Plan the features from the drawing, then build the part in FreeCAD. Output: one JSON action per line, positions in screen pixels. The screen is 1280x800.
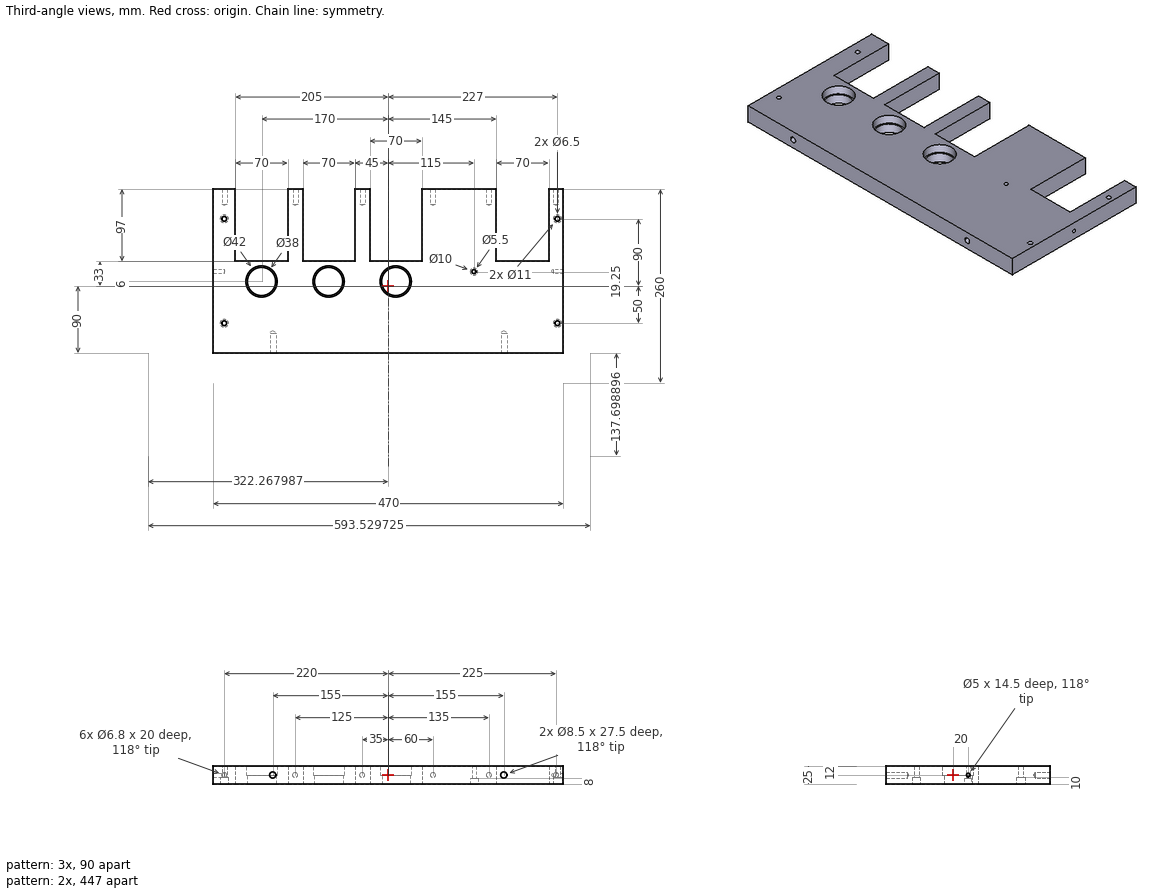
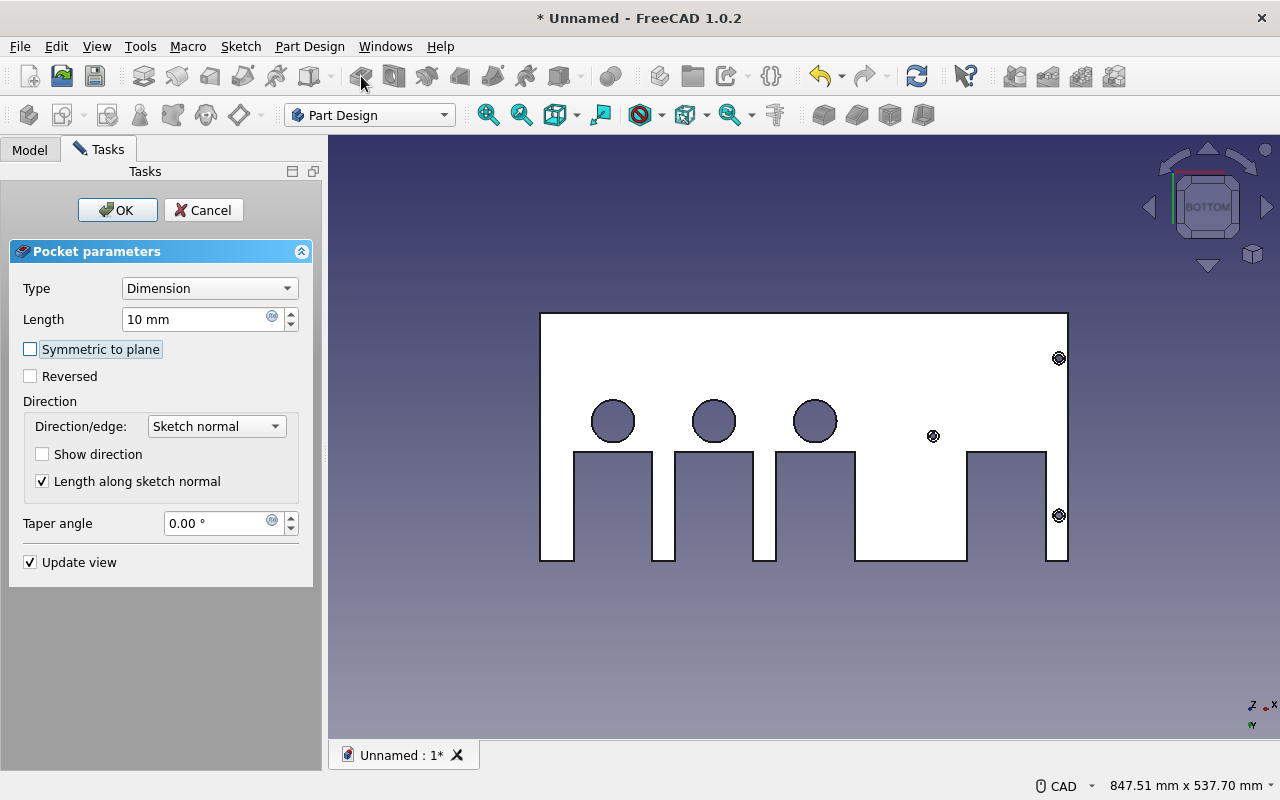
{"action": "left_click", "coordinate": [118, 210]}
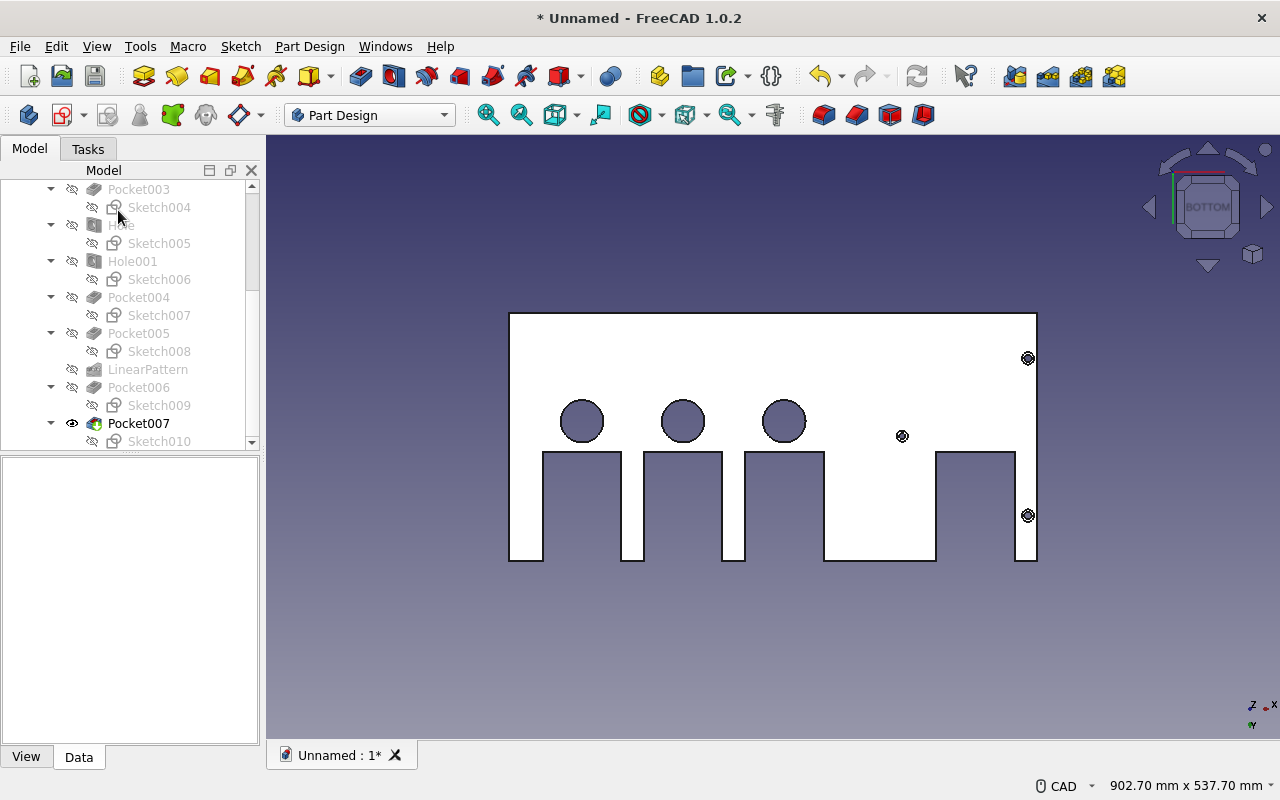
{"action": "left_click", "coordinate": [117, 387]}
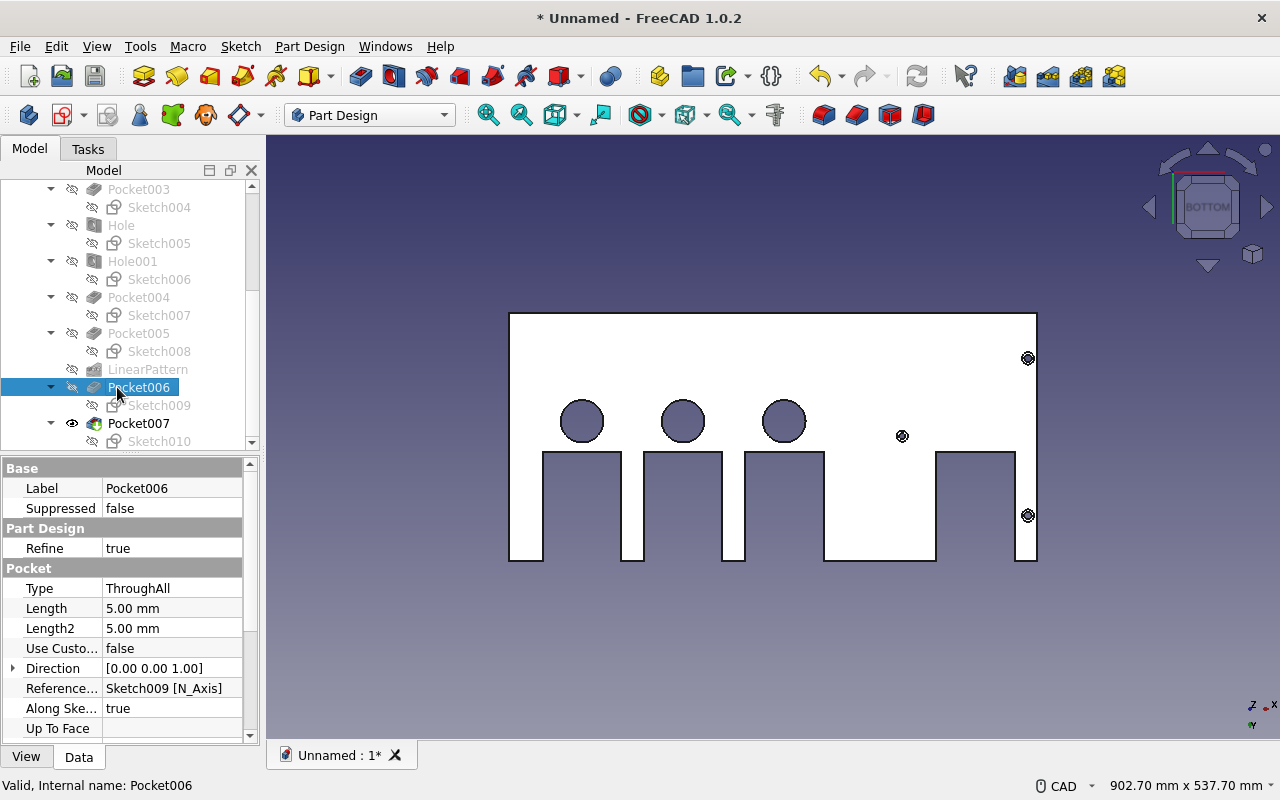
{"action": "left_click", "coordinate": [117, 423], "text": "ctrl"}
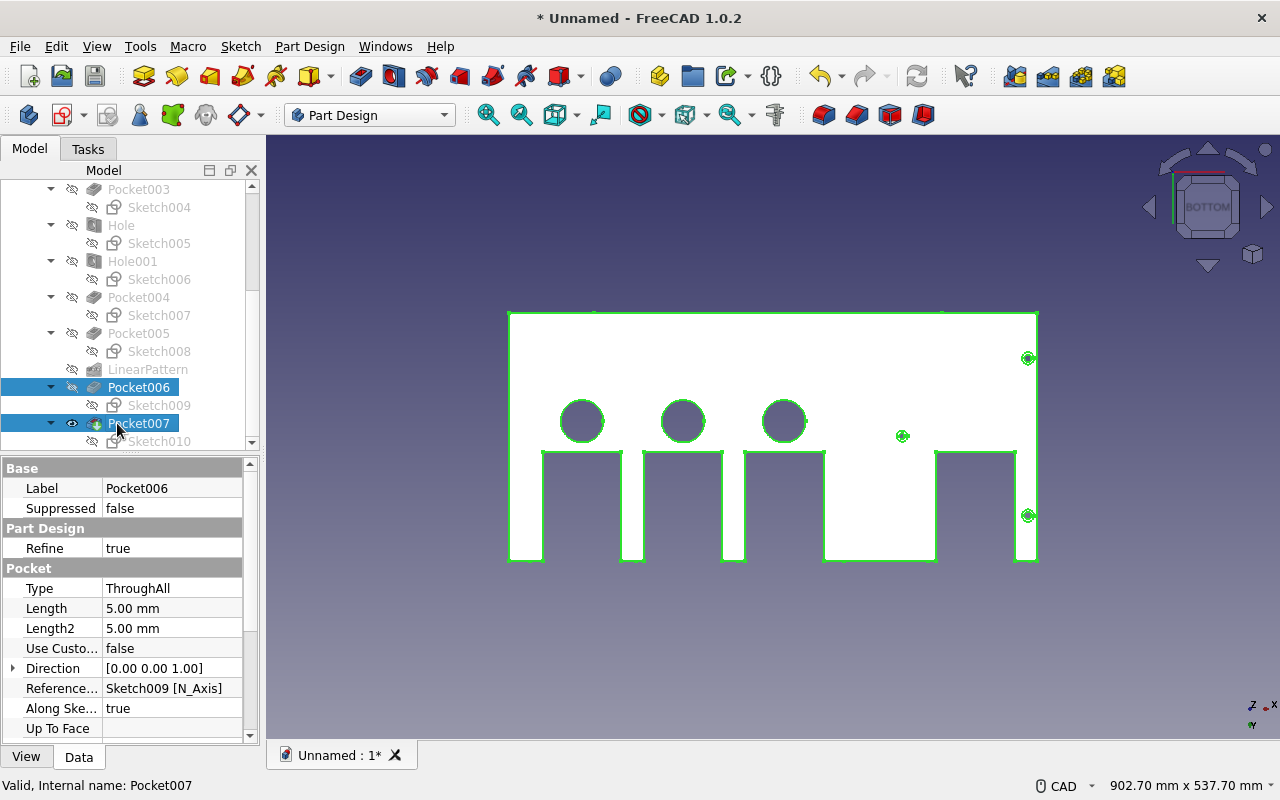
{"action": "left_click", "coordinate": [1048, 76]}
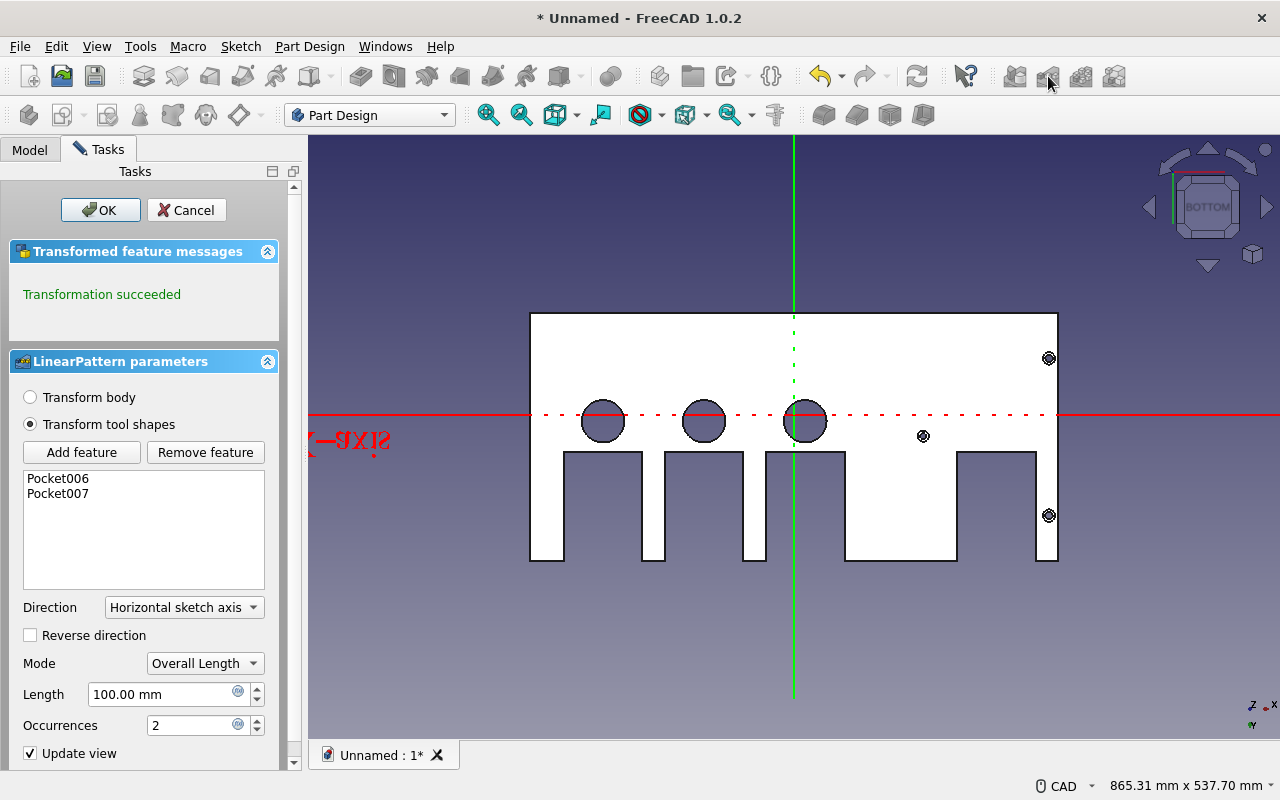
{"action": "left_click", "coordinate": [185, 608]}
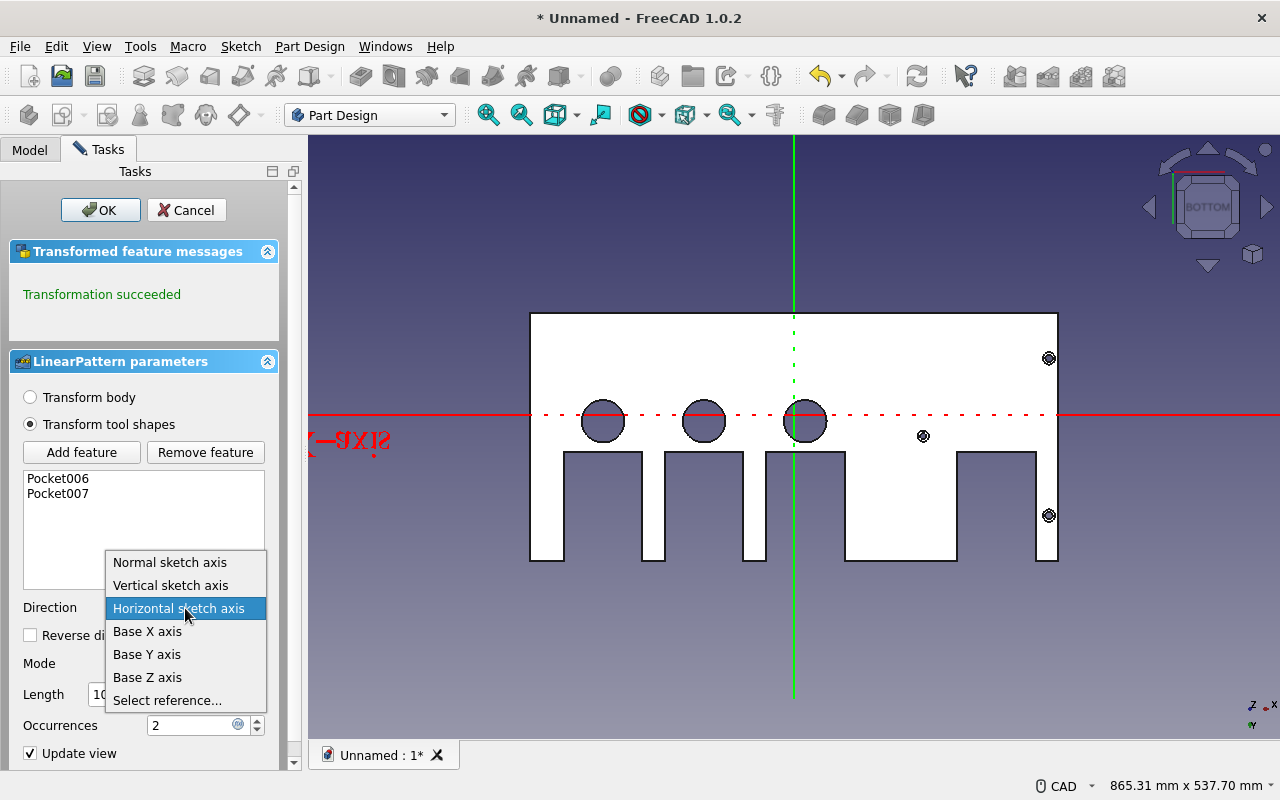
{"action": "left_click", "coordinate": [184, 632]}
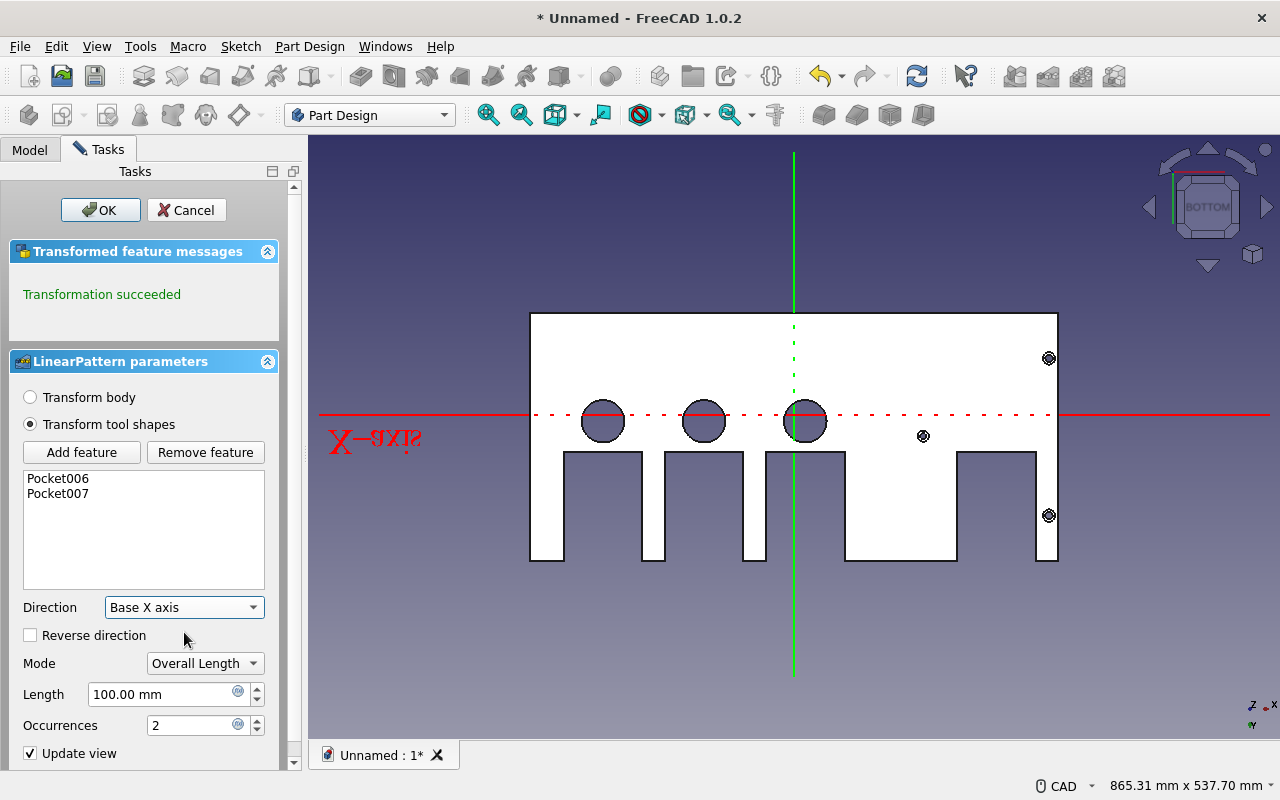
{"action": "left_click", "coordinate": [206, 664]}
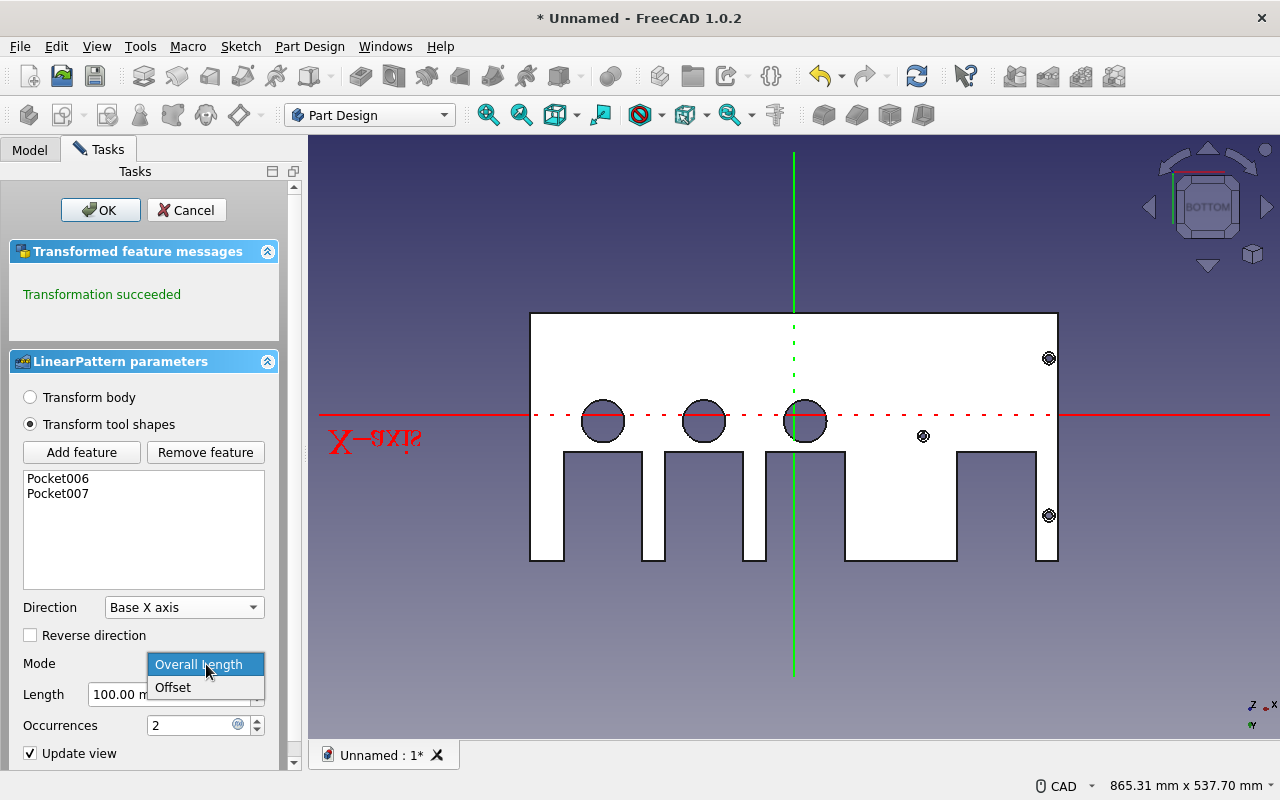
{"action": "left_click", "coordinate": [204, 688]}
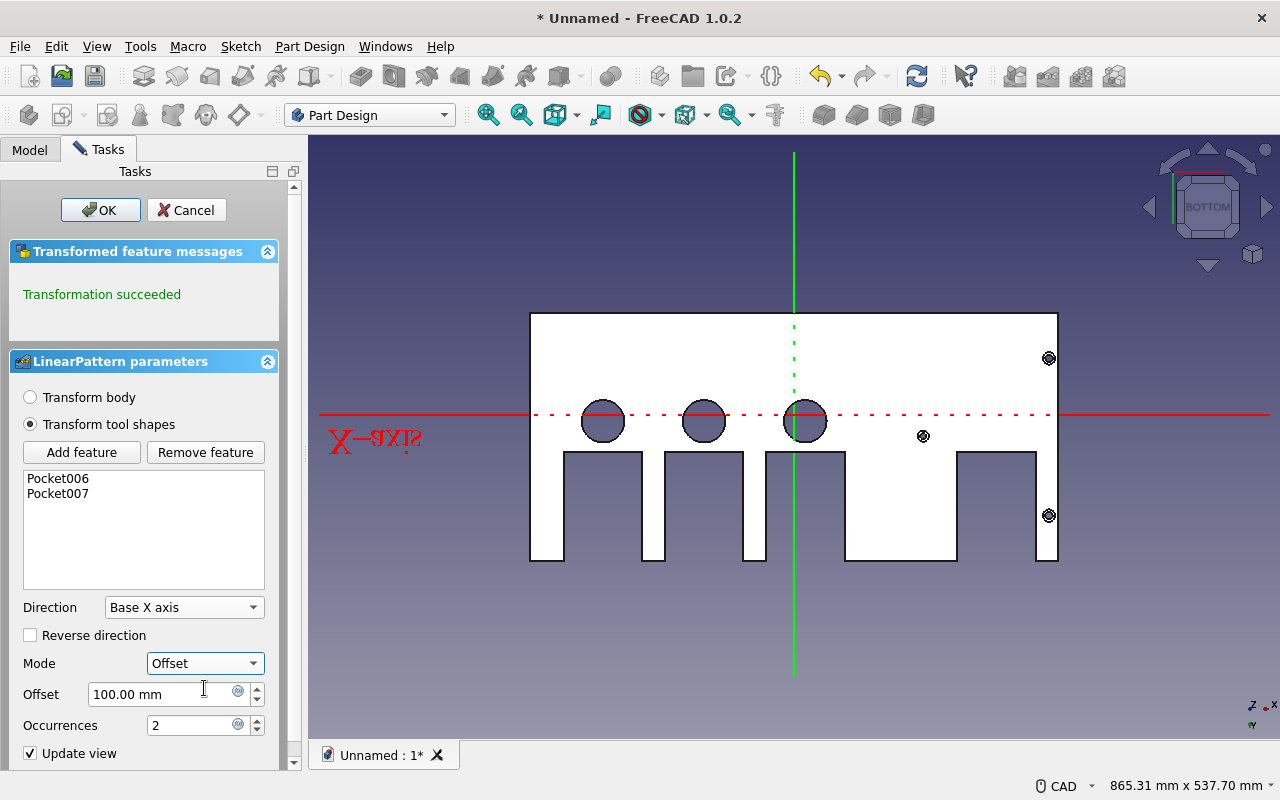
{"action": "triple_click", "coordinate": [170, 694]}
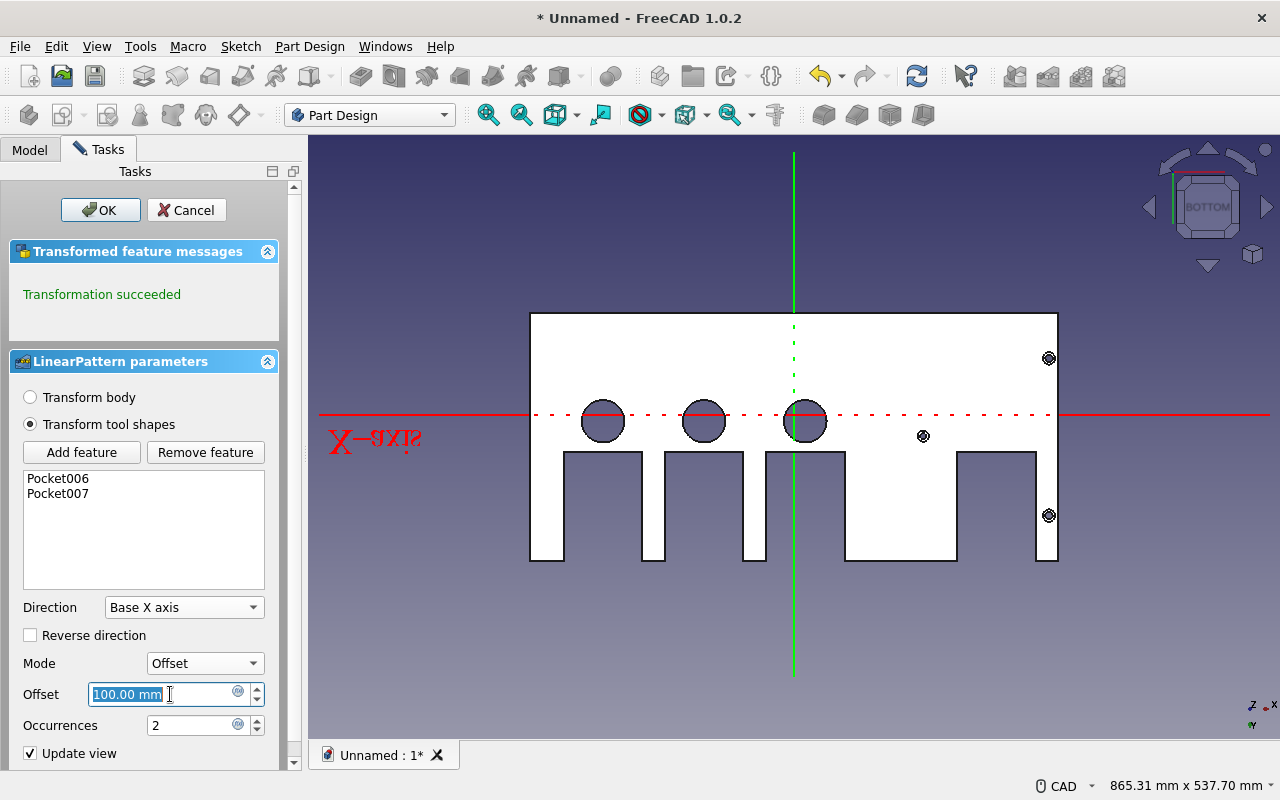
{"action": "type", "text": "447"}
{"action": "key", "text": "Tab"}